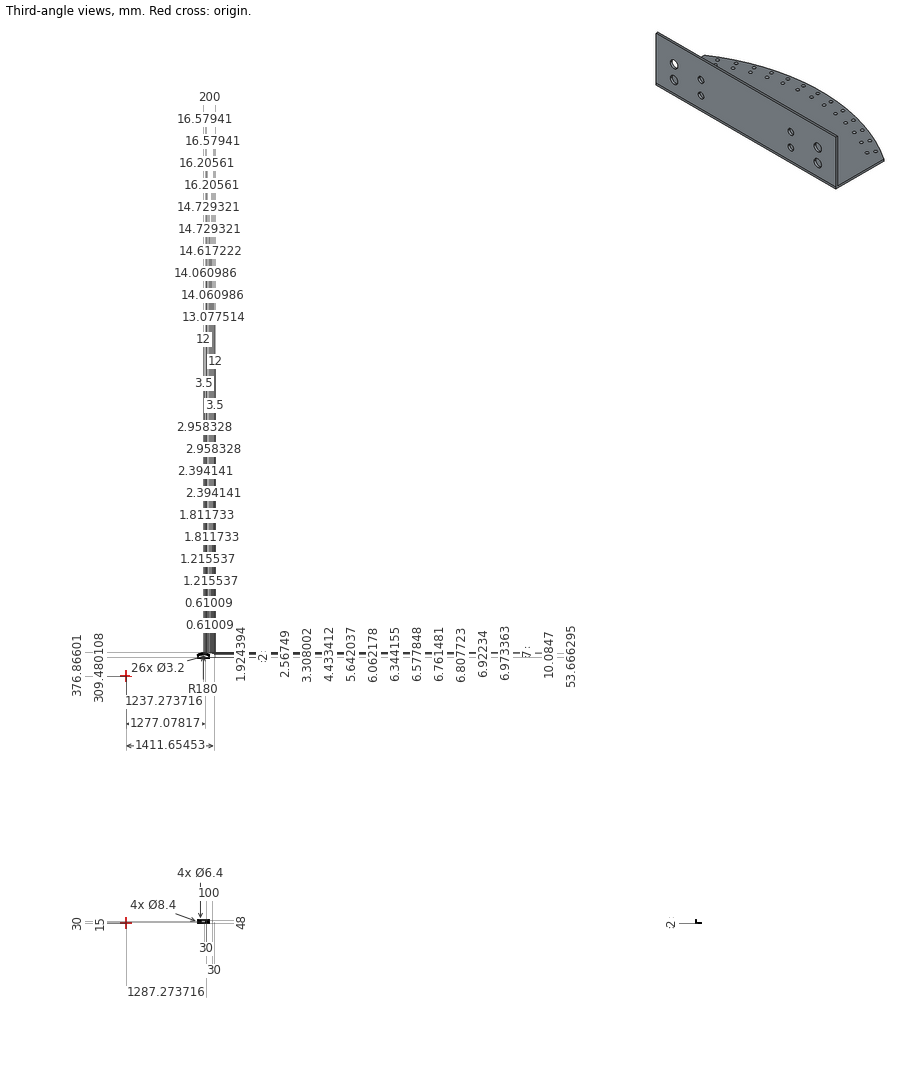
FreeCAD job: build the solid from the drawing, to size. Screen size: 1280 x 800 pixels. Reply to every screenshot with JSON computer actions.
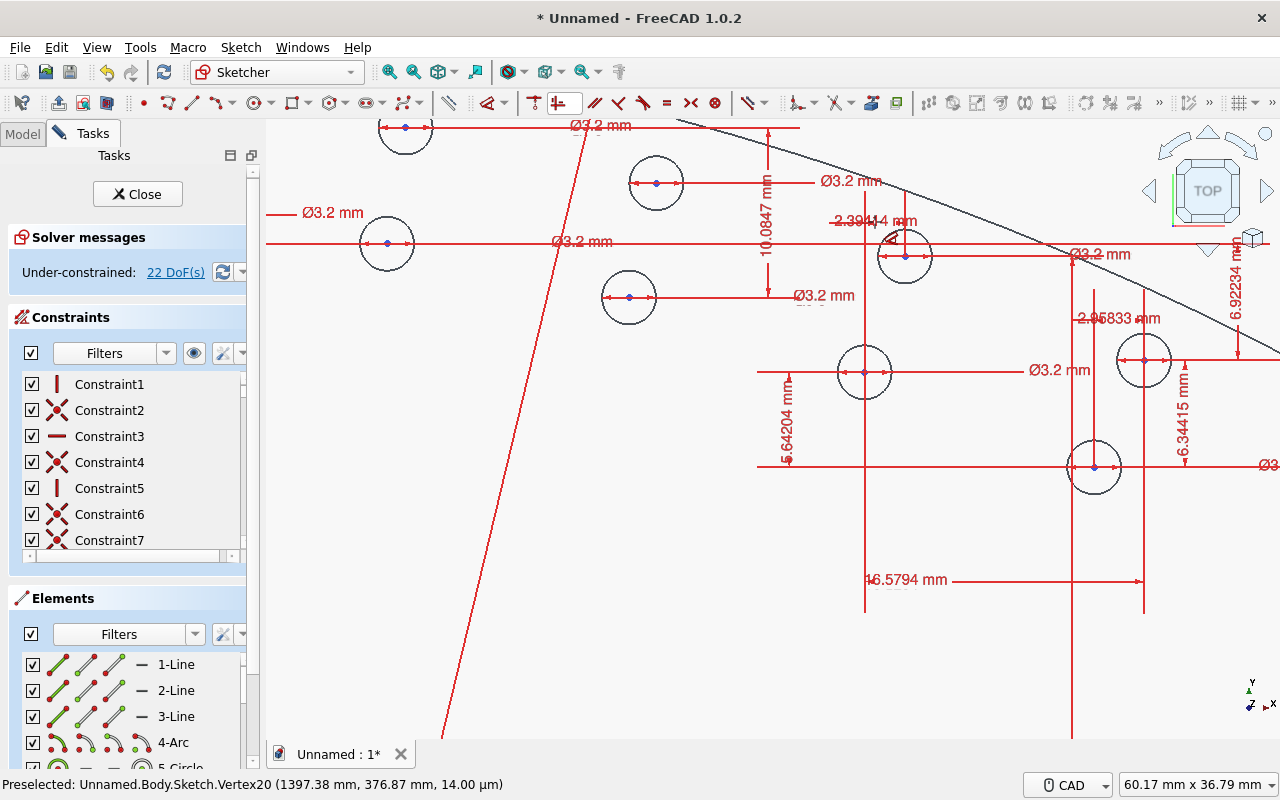
{"action": "left_click", "coordinate": [865, 372]}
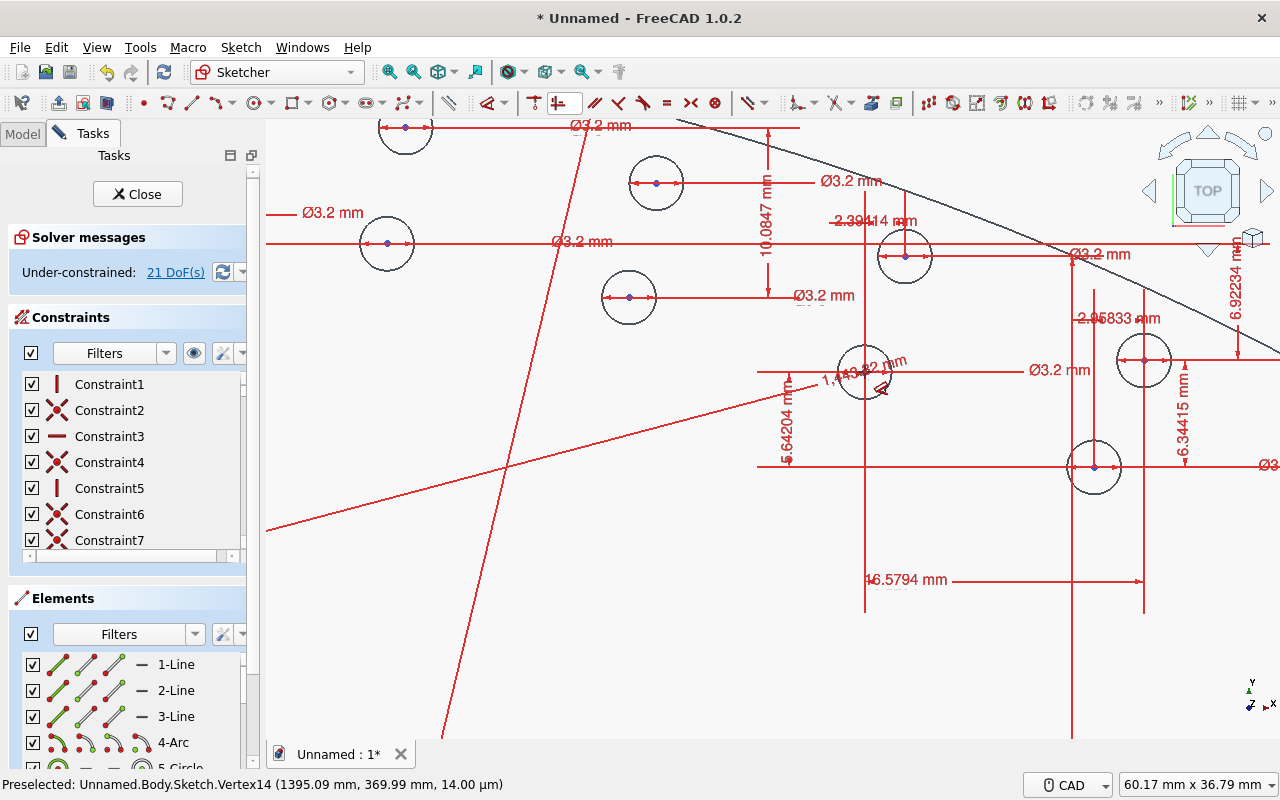
{"action": "left_click", "coordinate": [905, 256]}
{"action": "left_click", "coordinate": [939, 314]}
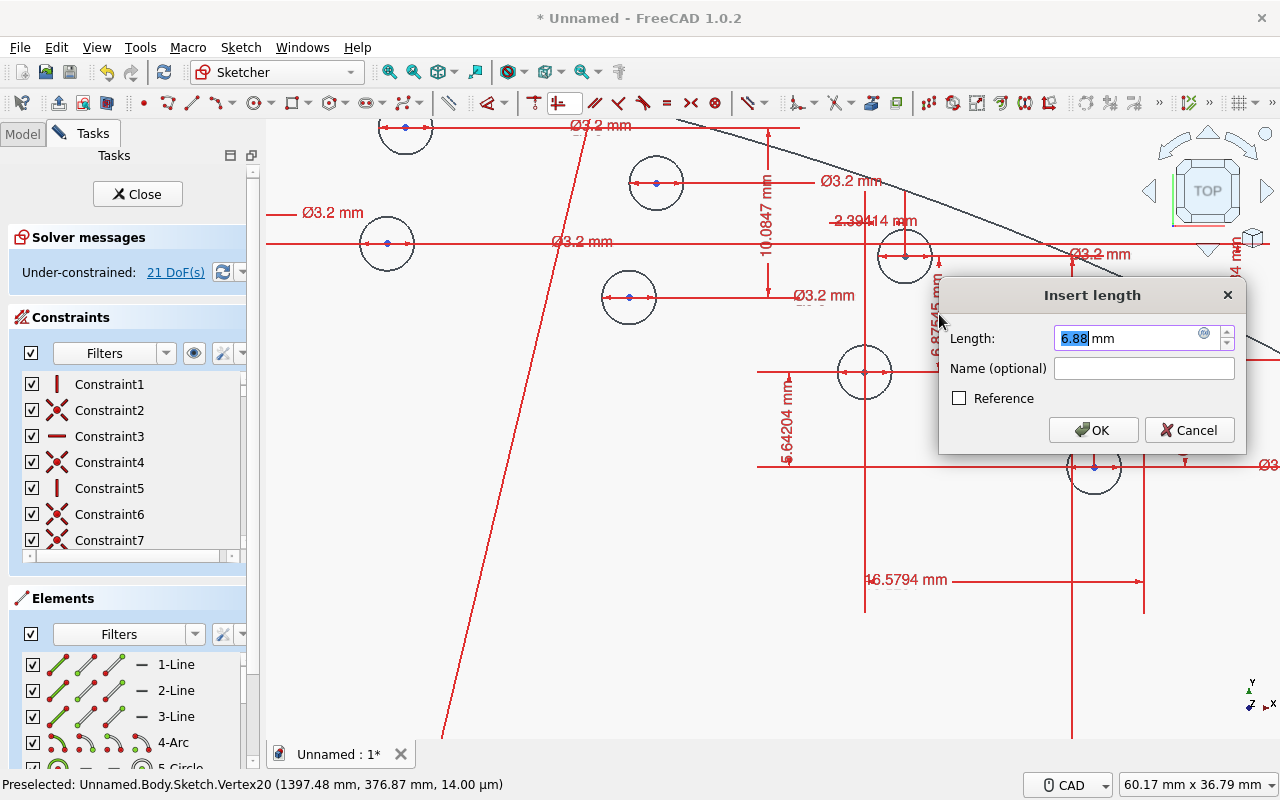
{"action": "type", "text": "6.577848"}
{"action": "key", "text": "Return"}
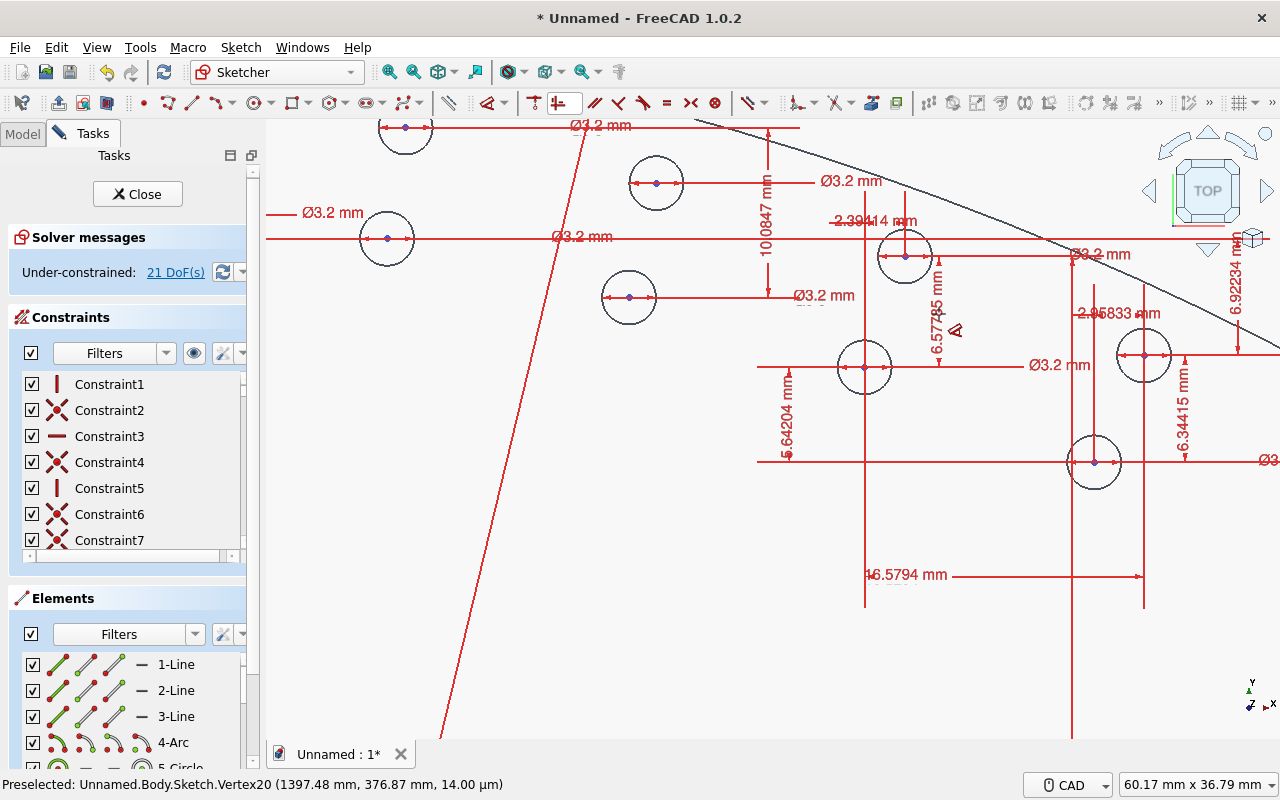
{"action": "left_click", "coordinate": [865, 367]}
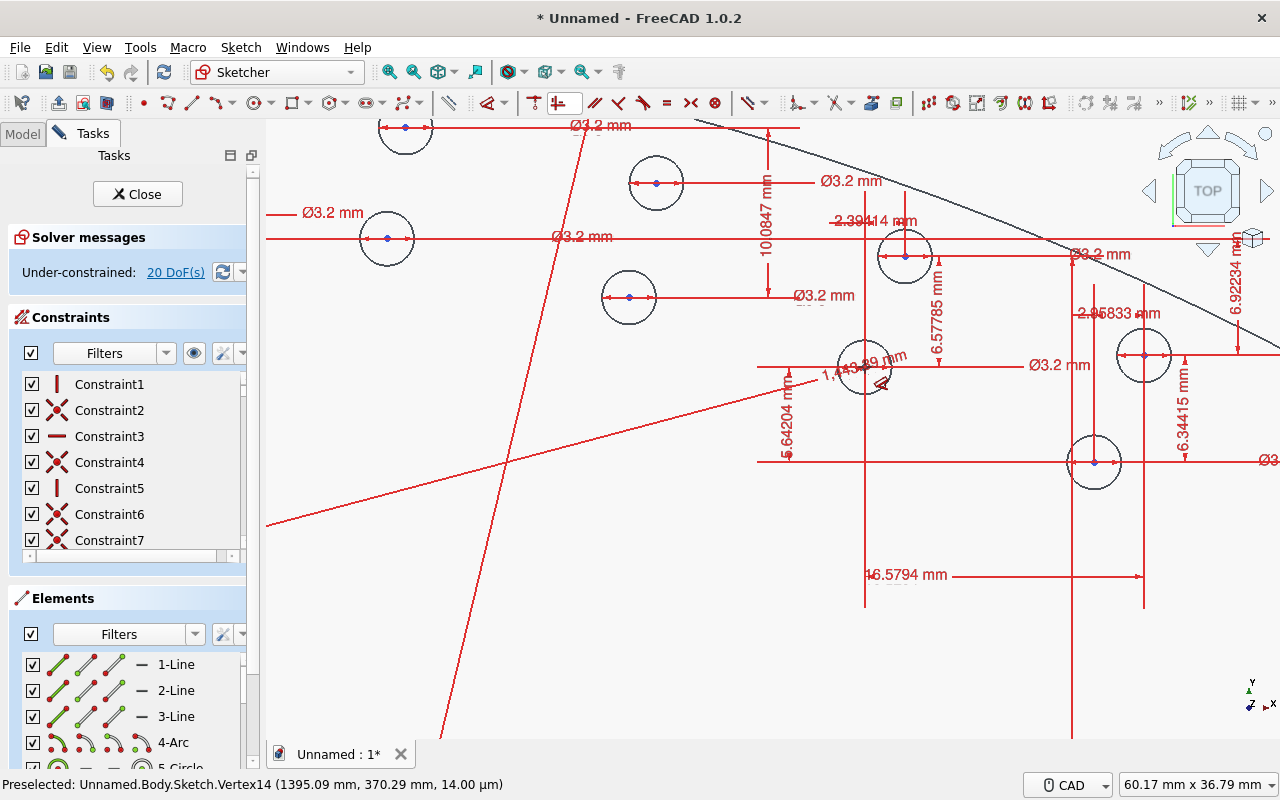
{"action": "left_click", "coordinate": [629, 298]}
{"action": "left_click", "coordinate": [595, 332]}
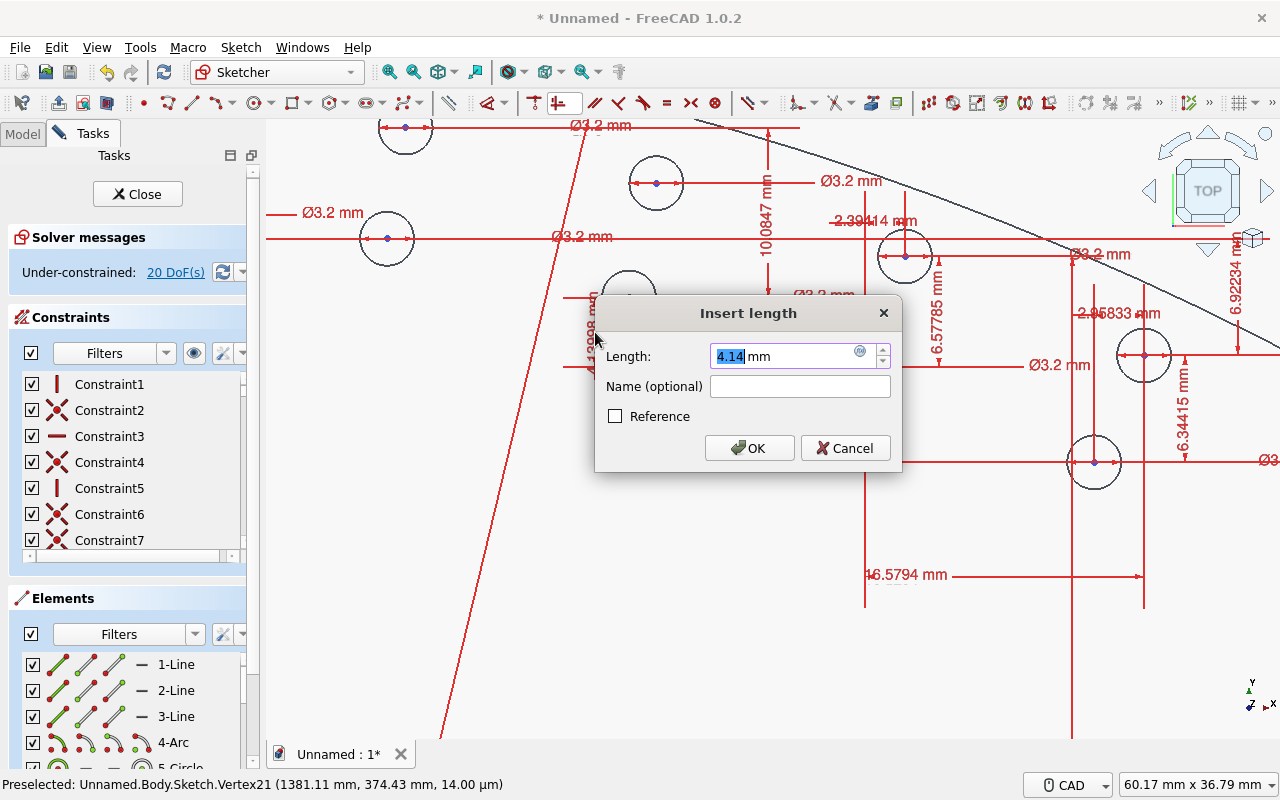
{"action": "type", "text": "4.433412"}
{"action": "key", "text": "Return"}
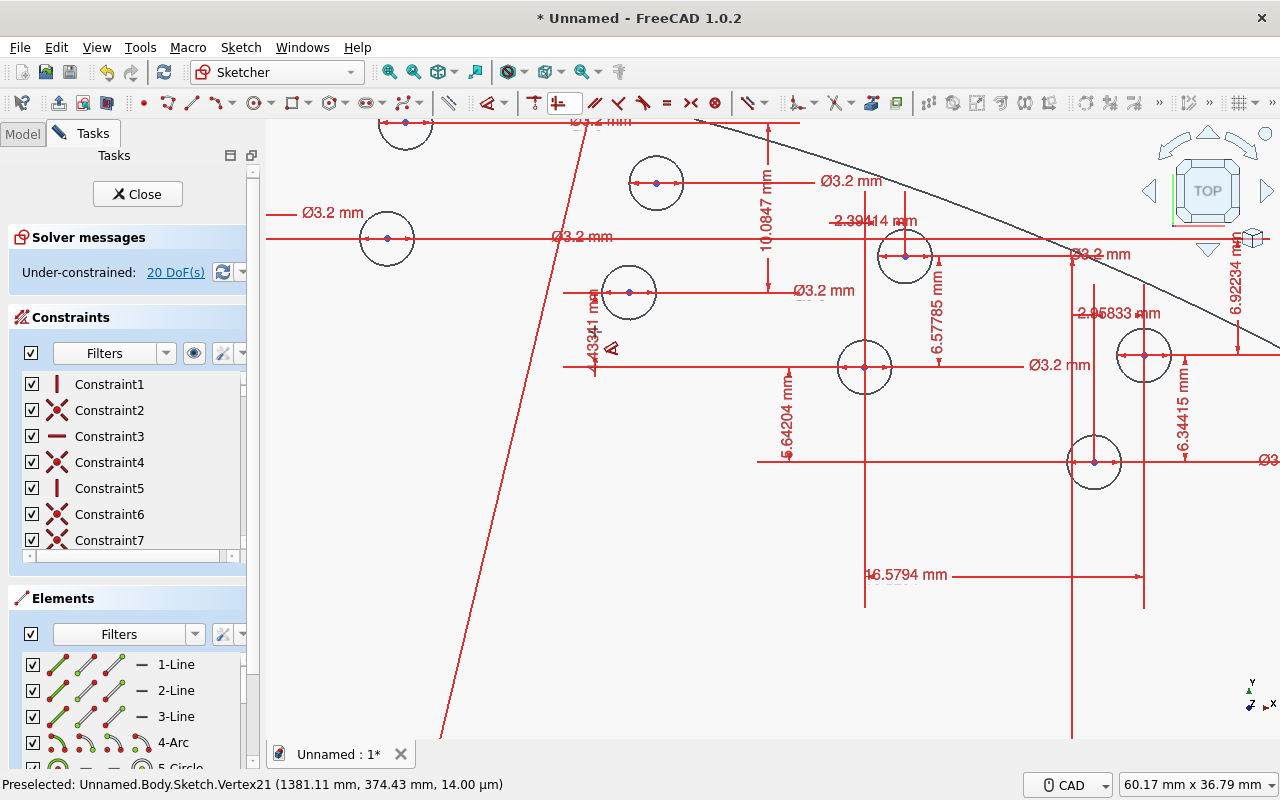
{"action": "scroll", "coordinate": [387, 239], "scroll_direction": "up", "scroll_amount": 2}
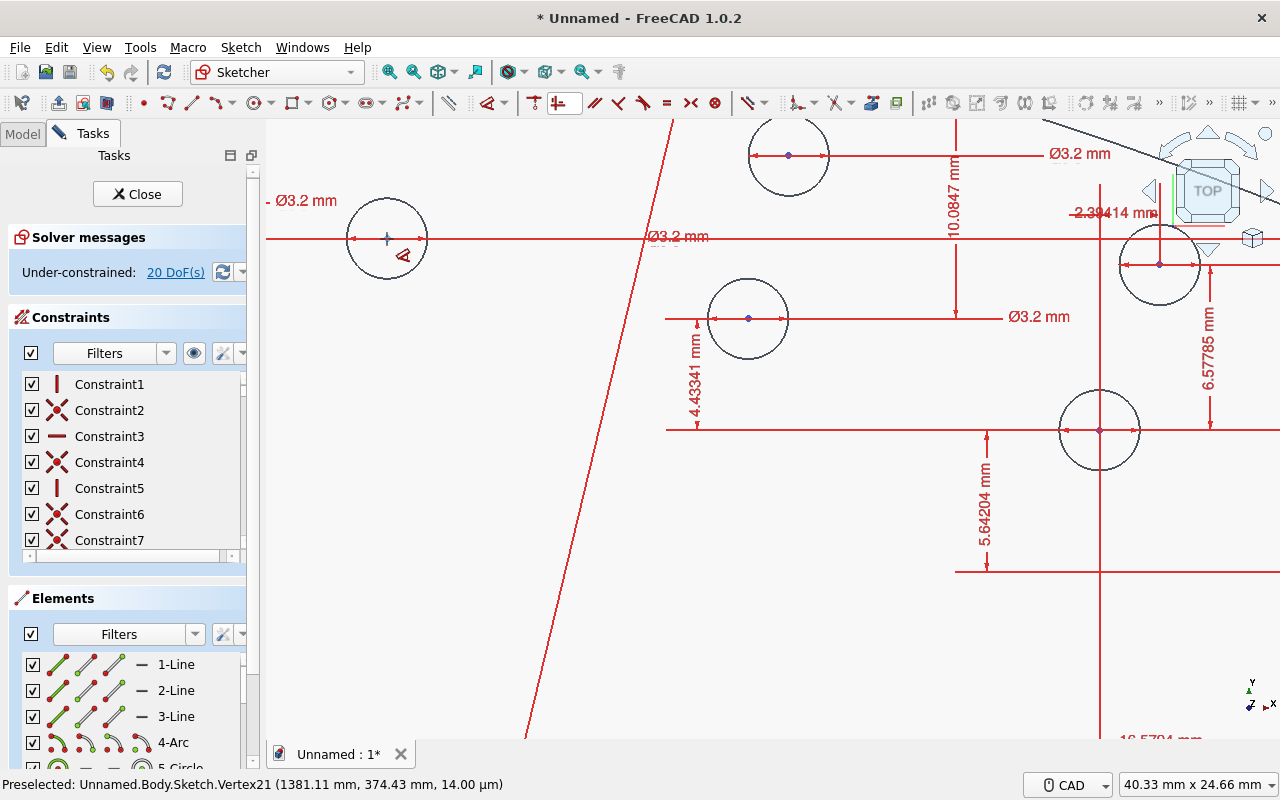
{"action": "left_click", "coordinate": [387, 239]}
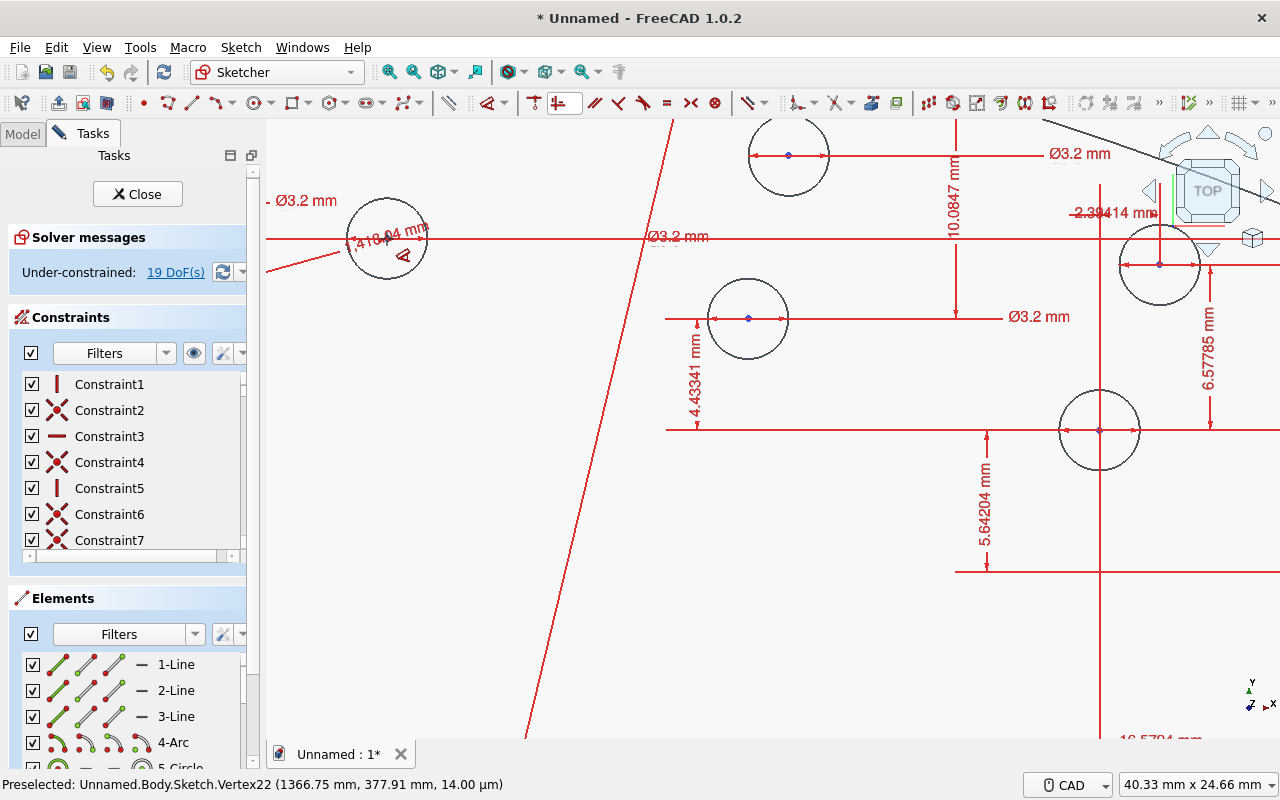
{"action": "scroll", "coordinate": [836, 364], "scroll_direction": "down", "scroll_amount": 11}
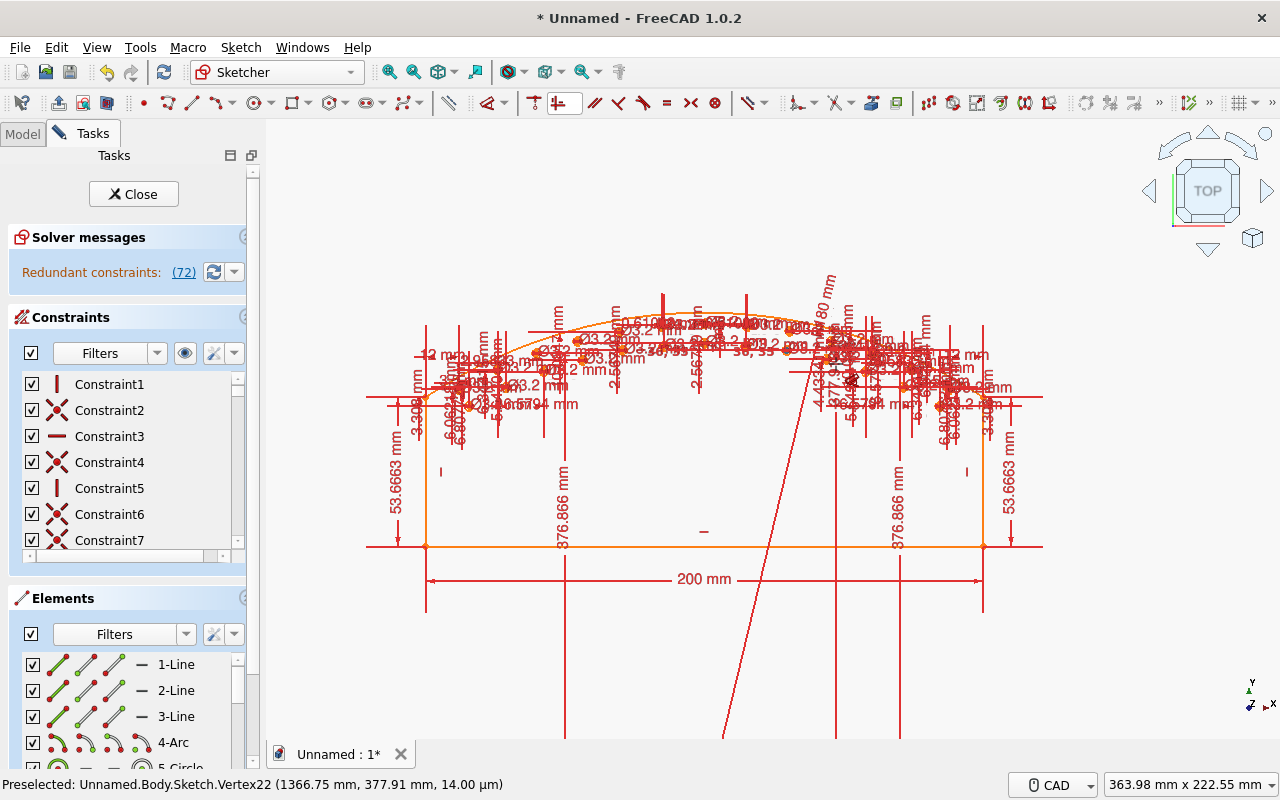
{"action": "scroll", "coordinate": [746, 346], "scroll_direction": "up", "scroll_amount": 11}